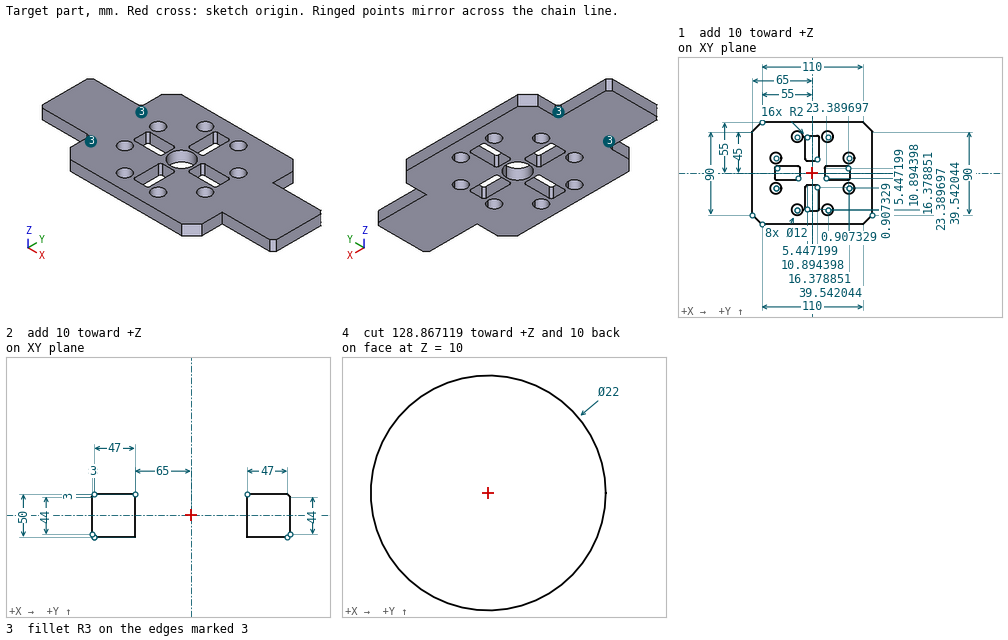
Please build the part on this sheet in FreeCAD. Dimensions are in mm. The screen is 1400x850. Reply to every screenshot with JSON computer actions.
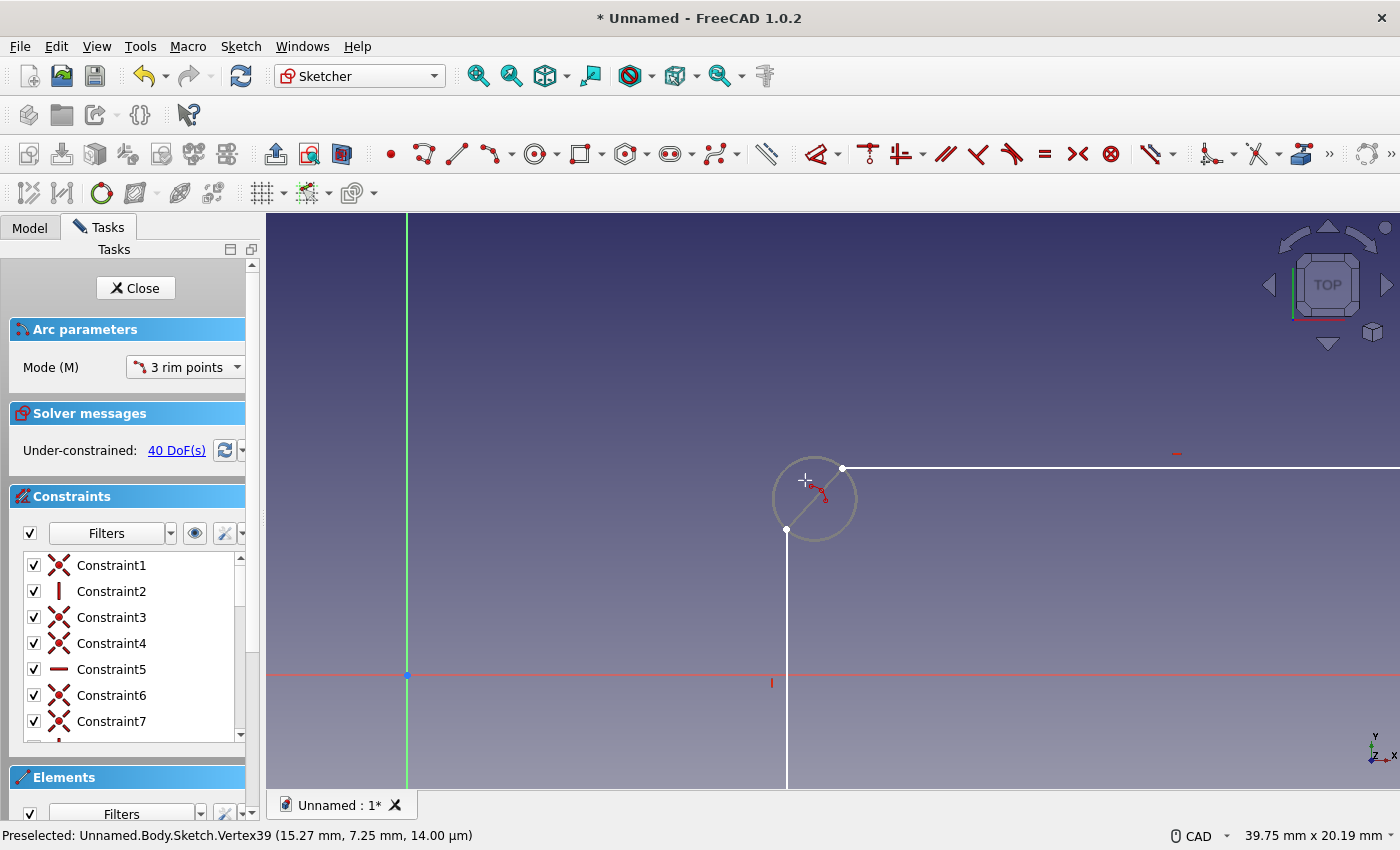
{"action": "left_click", "coordinate": [802, 479]}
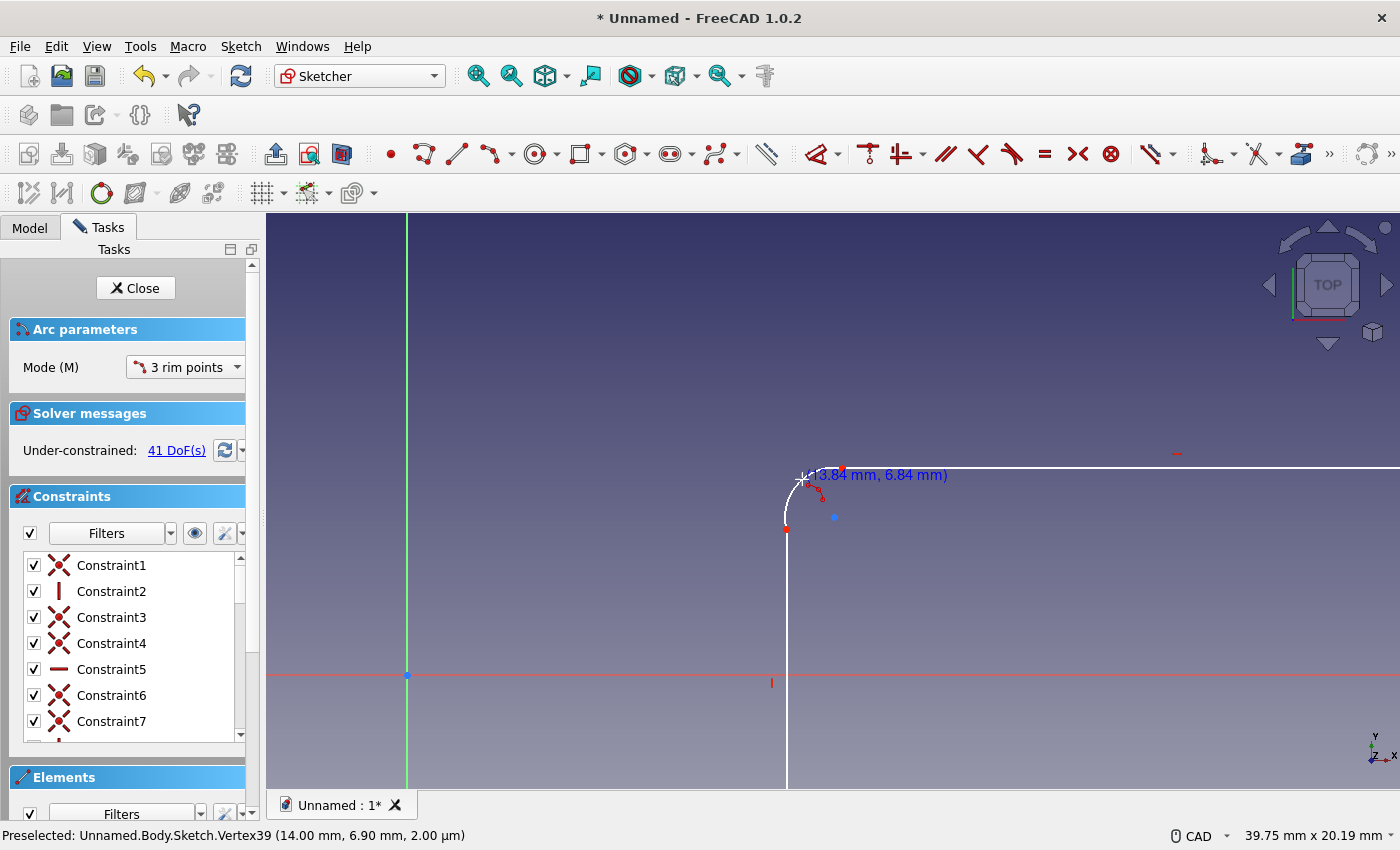
{"action": "scroll", "coordinate": [809, 479], "scroll_direction": "down", "scroll_amount": 11}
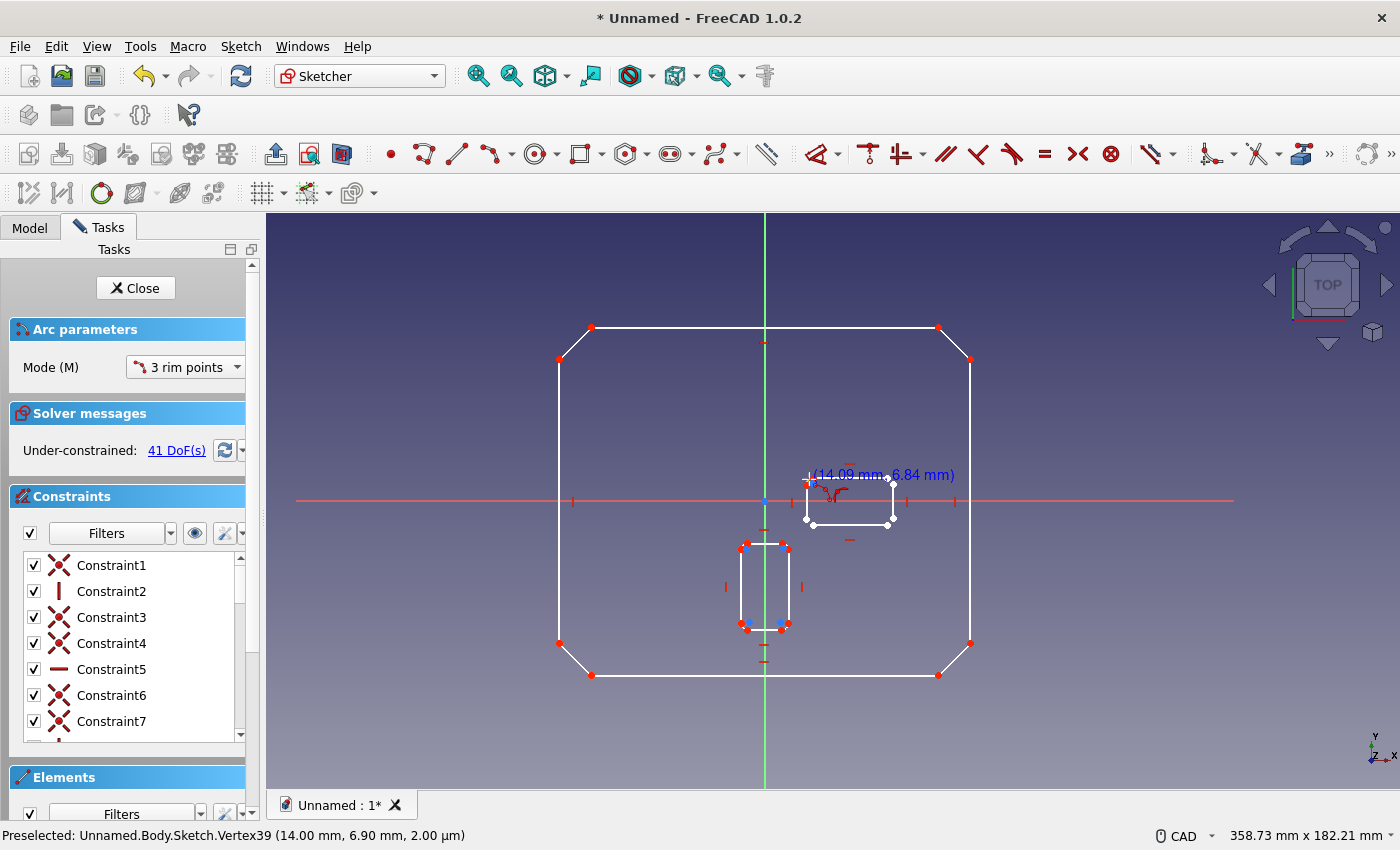
{"action": "scroll", "coordinate": [887, 478], "scroll_direction": "up", "scroll_amount": 3}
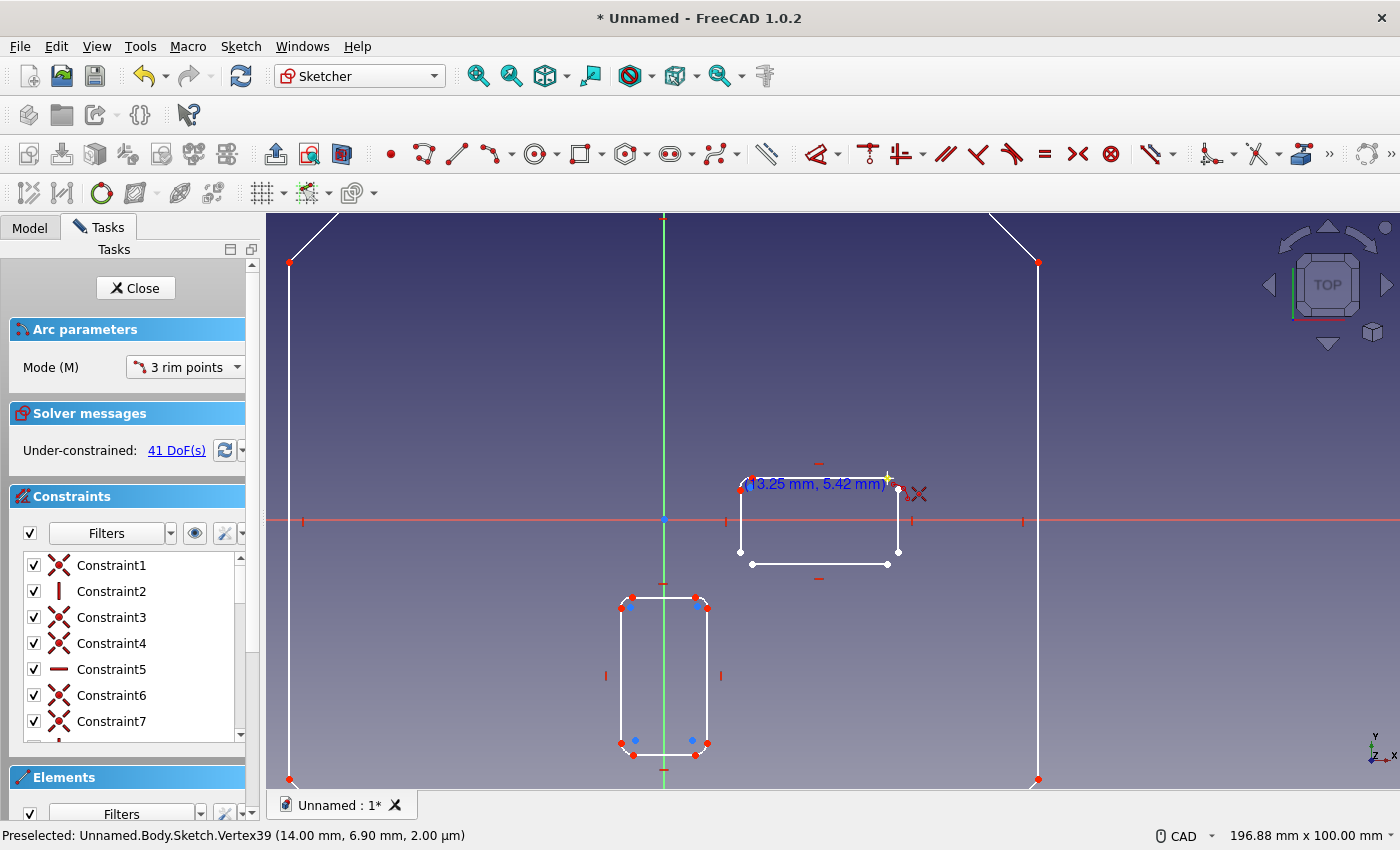
{"action": "left_click", "coordinate": [887, 478]}
{"action": "left_click", "coordinate": [898, 489]}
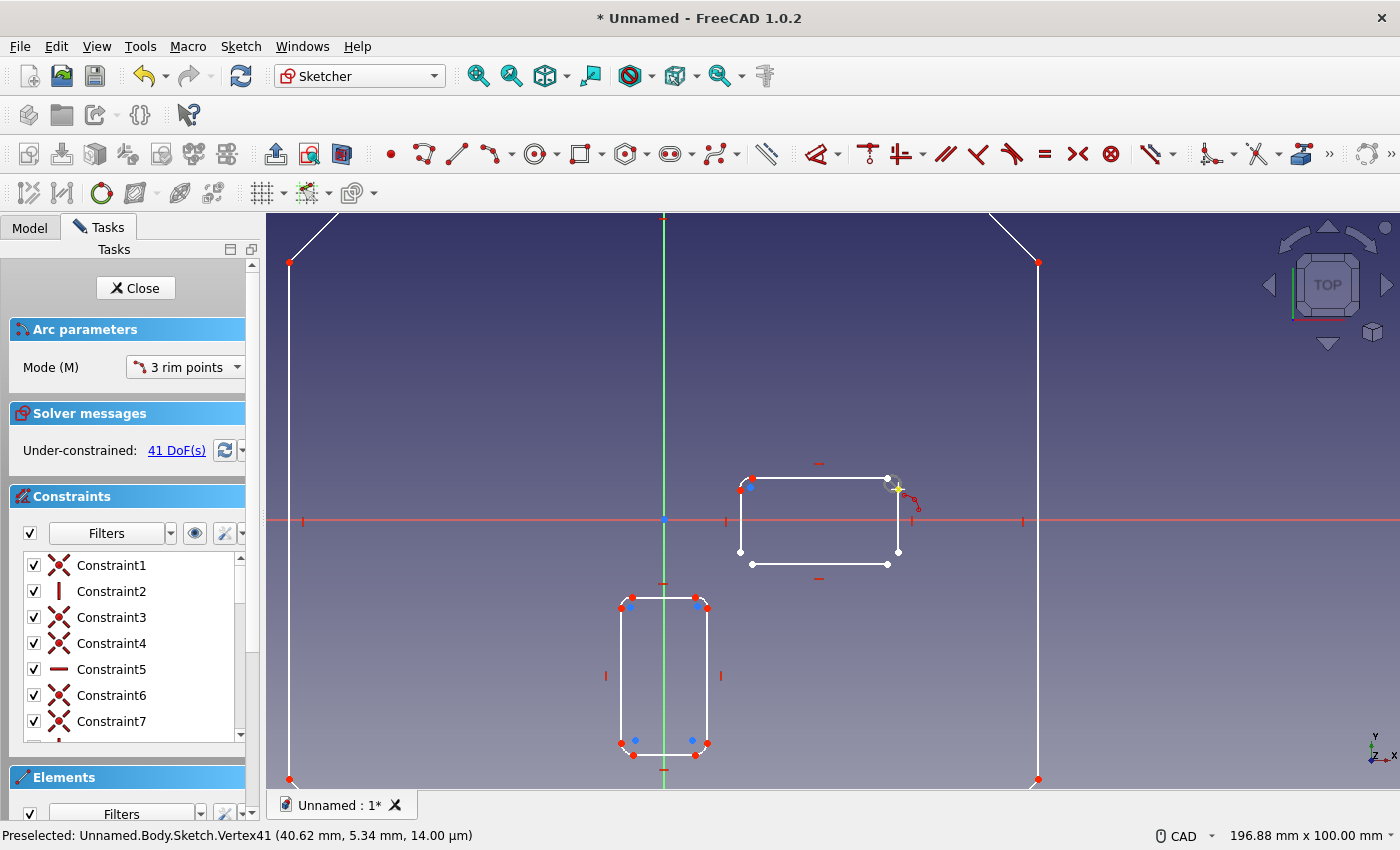
{"action": "scroll", "coordinate": [895, 480], "scroll_direction": "up", "scroll_amount": 8}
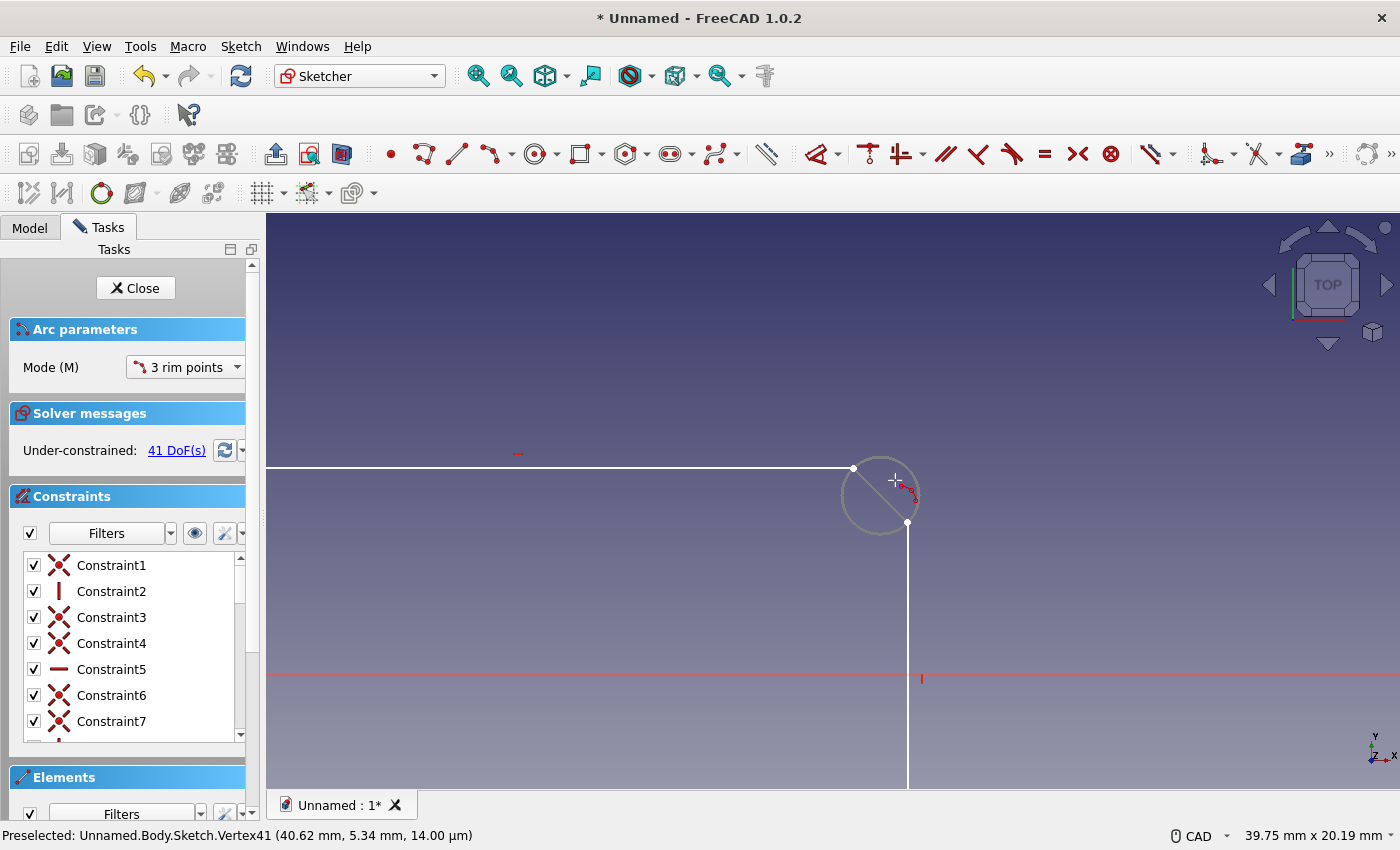
{"action": "left_click", "coordinate": [891, 480]}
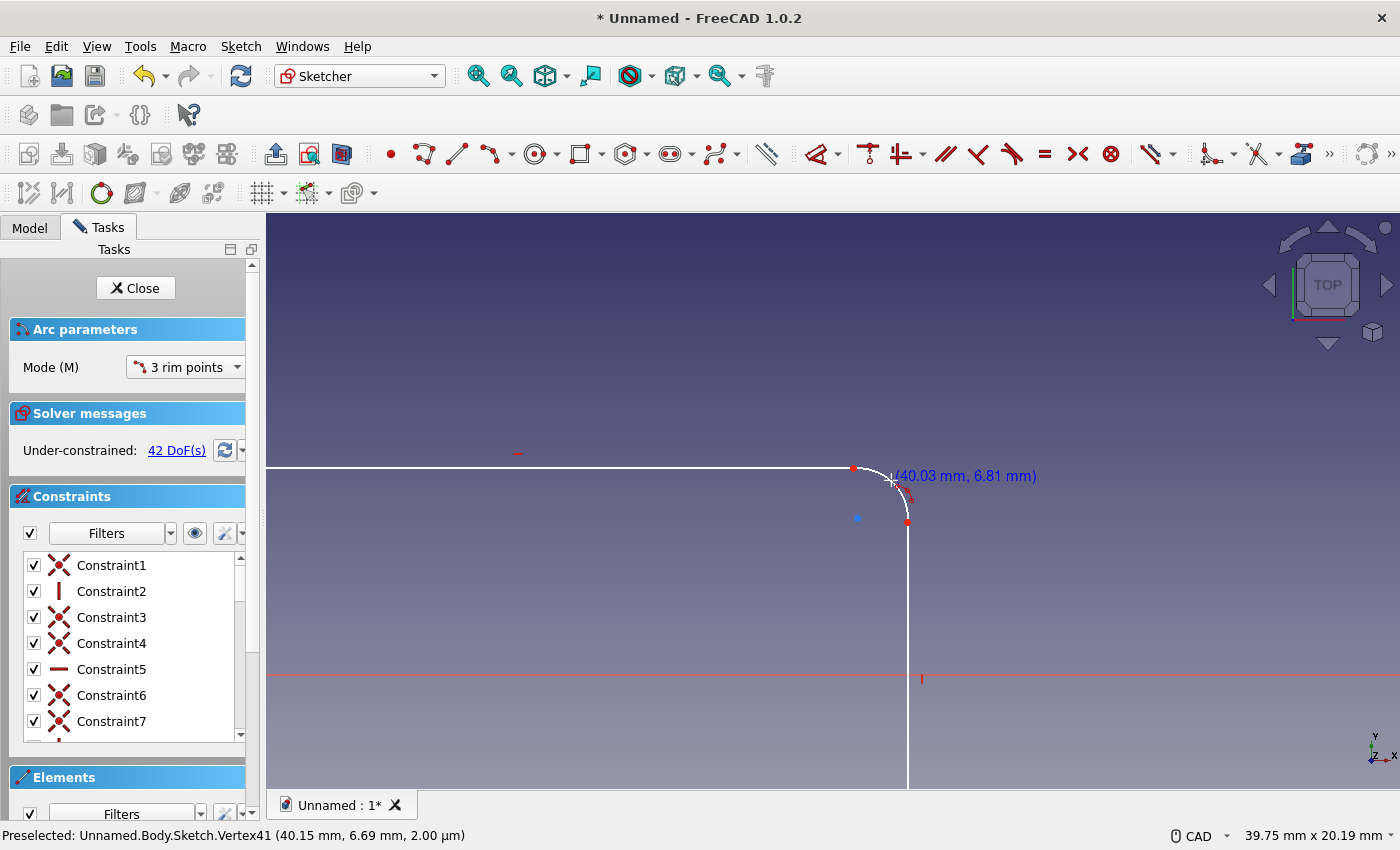
{"action": "scroll", "coordinate": [891, 479], "scroll_direction": "down", "scroll_amount": 11}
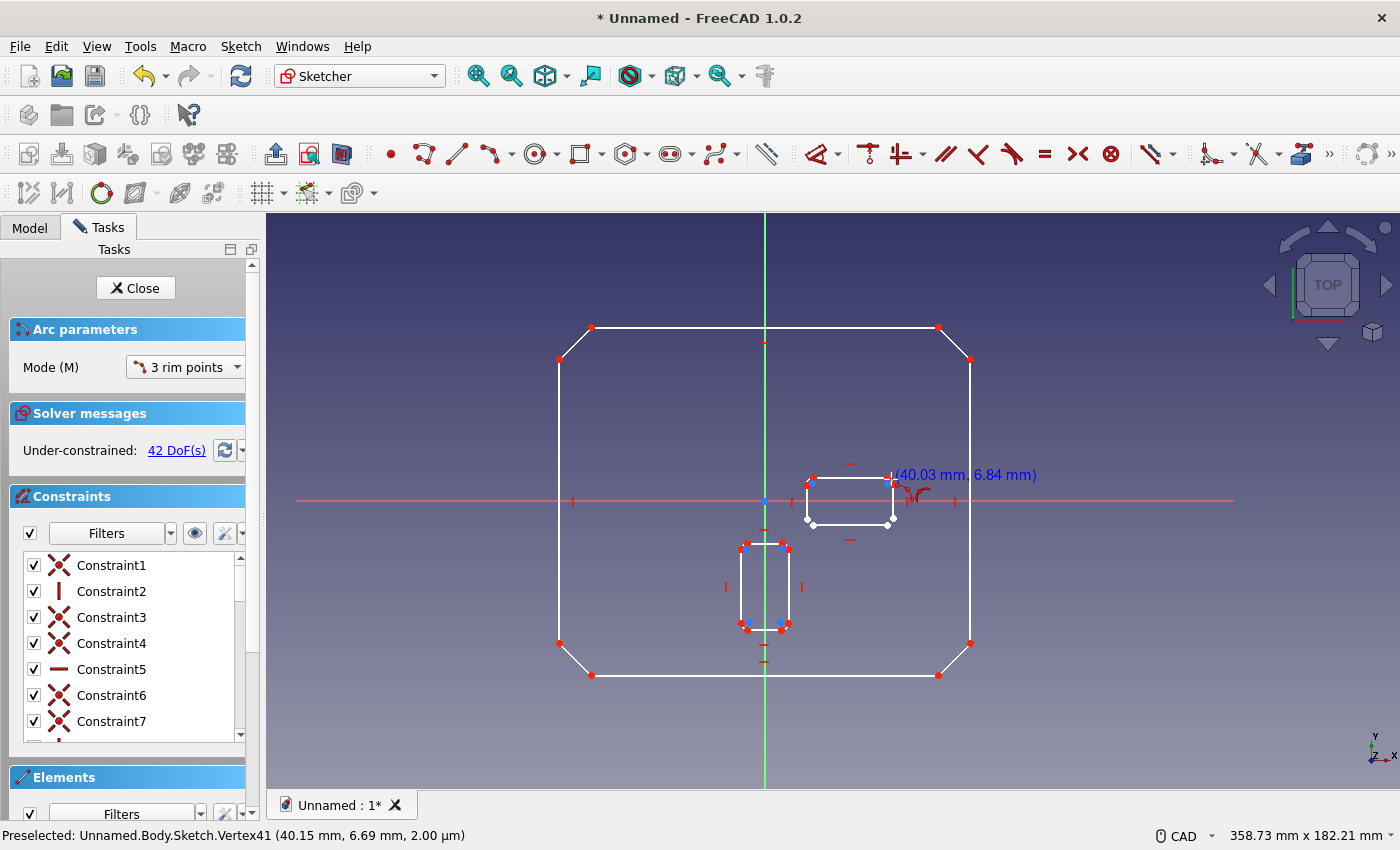
{"action": "scroll", "coordinate": [893, 518], "scroll_direction": "up", "scroll_amount": 3}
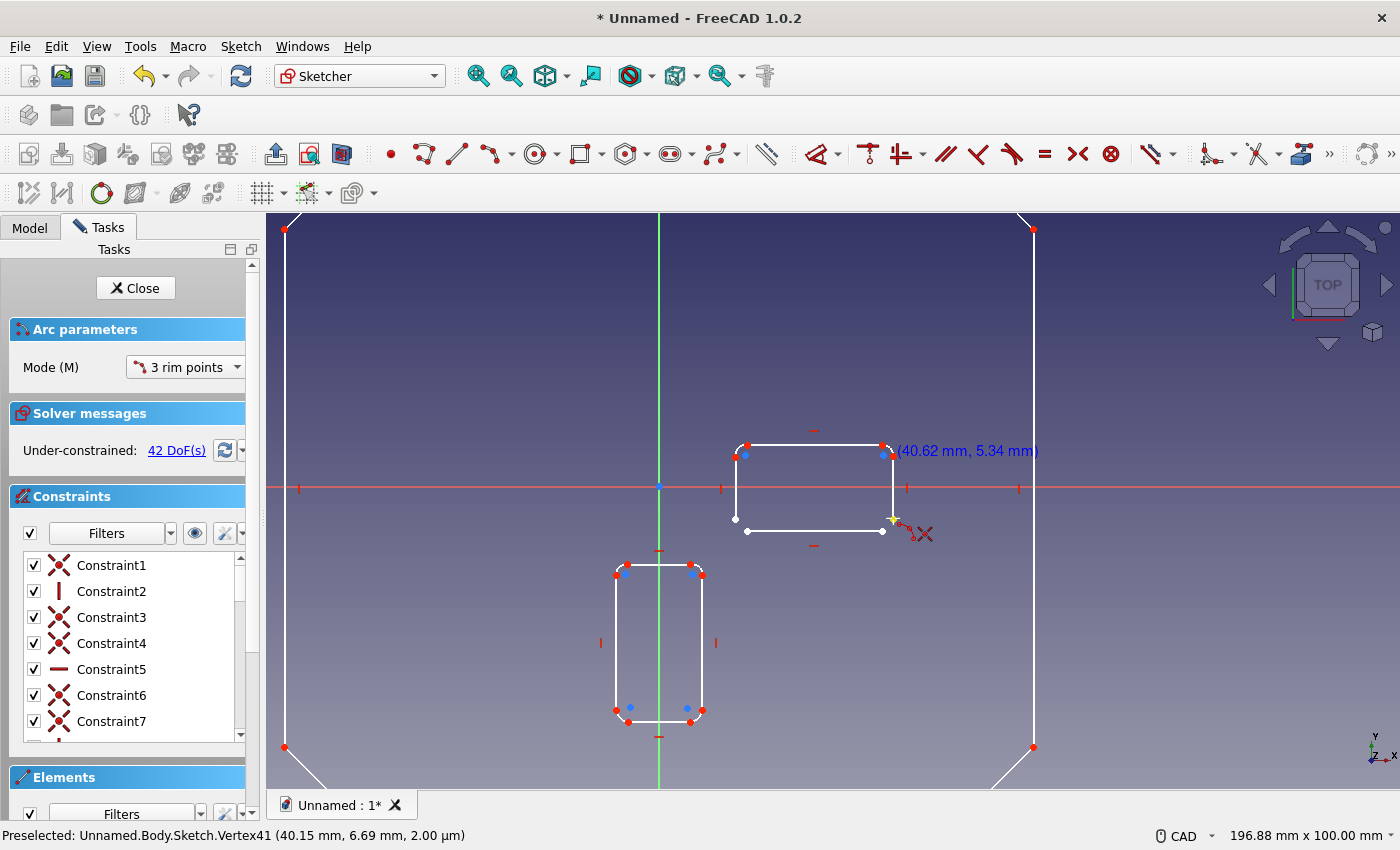
{"action": "left_click", "coordinate": [893, 519]}
{"action": "left_click", "coordinate": [882, 531]}